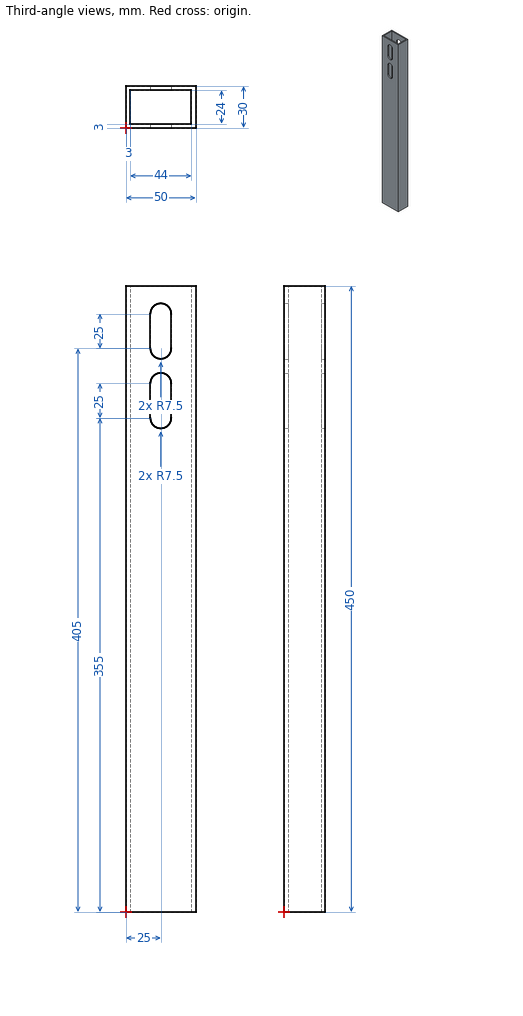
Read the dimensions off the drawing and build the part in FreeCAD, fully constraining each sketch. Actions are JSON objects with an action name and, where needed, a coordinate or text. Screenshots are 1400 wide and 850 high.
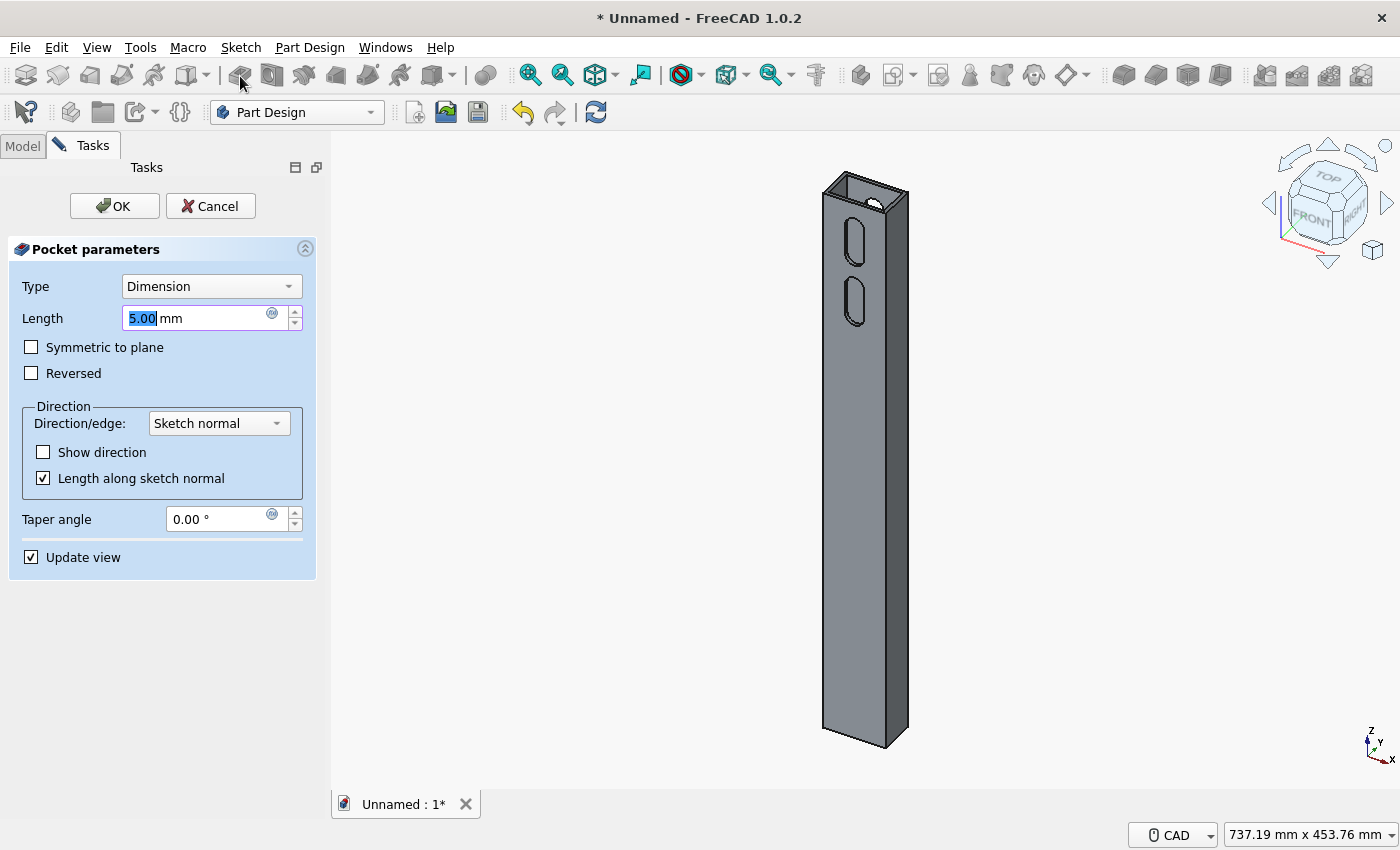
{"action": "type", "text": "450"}
{"action": "key", "text": "Tab"}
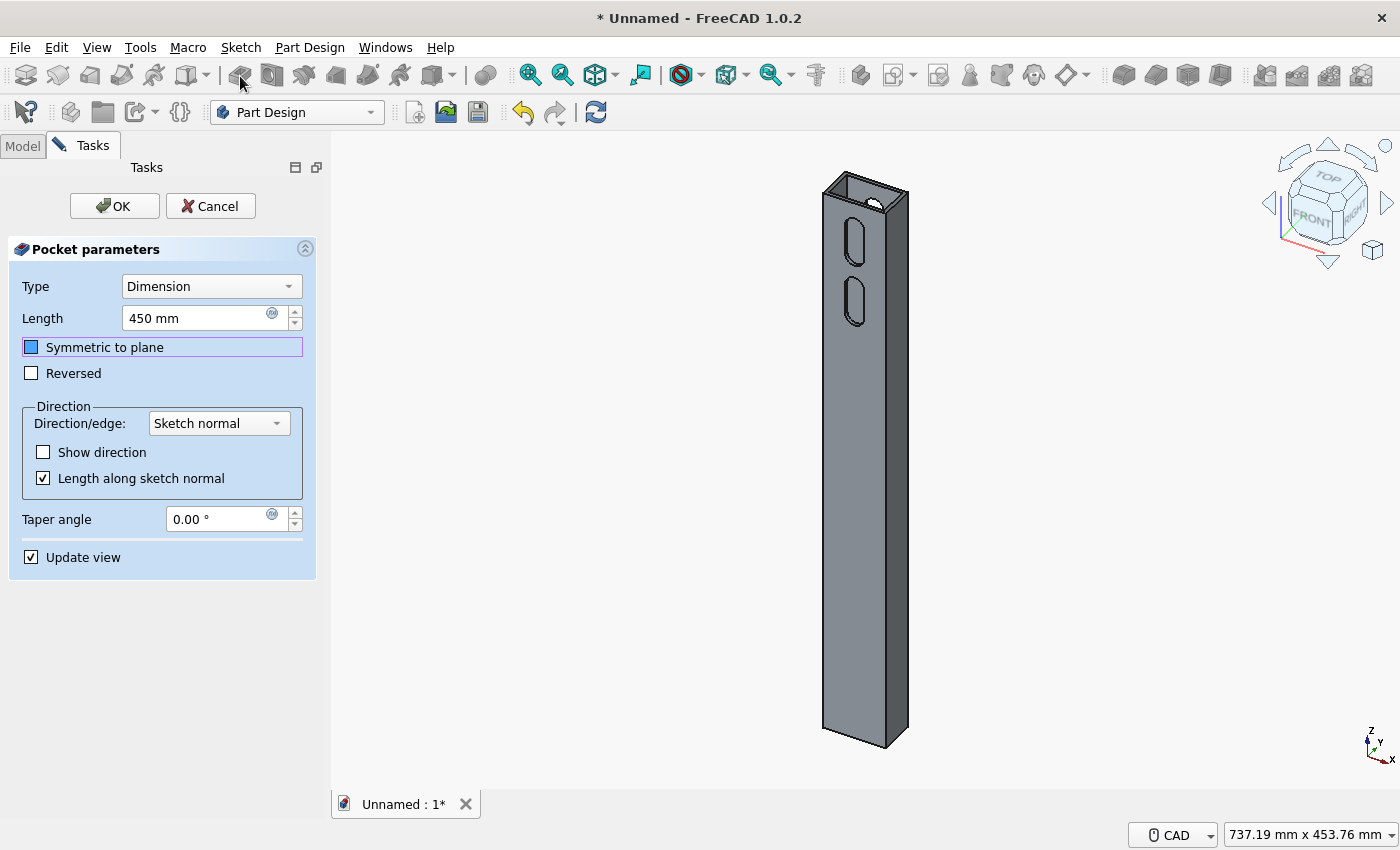
{"action": "left_click", "coordinate": [115, 206]}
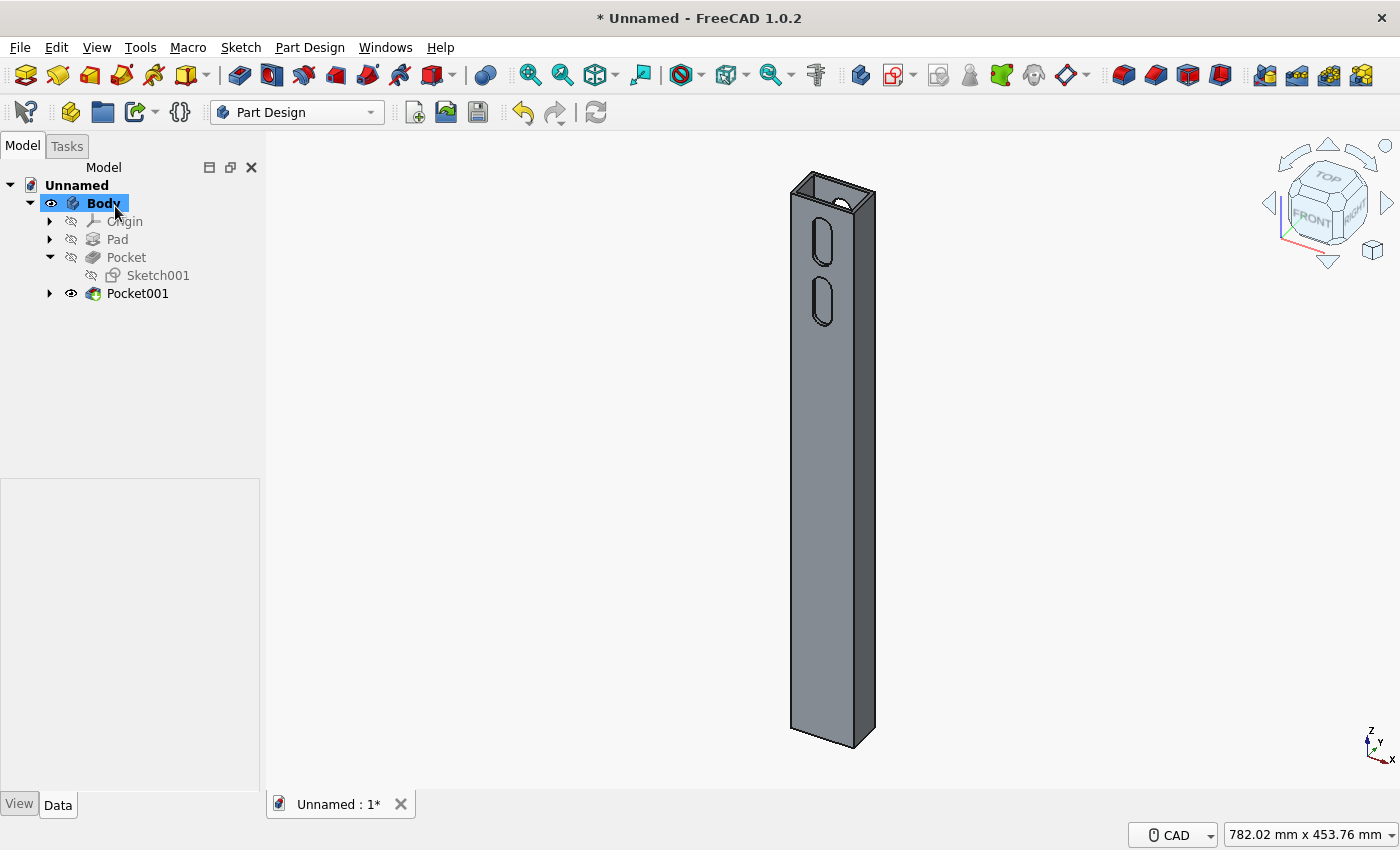
{"action": "key", "text": "0"}